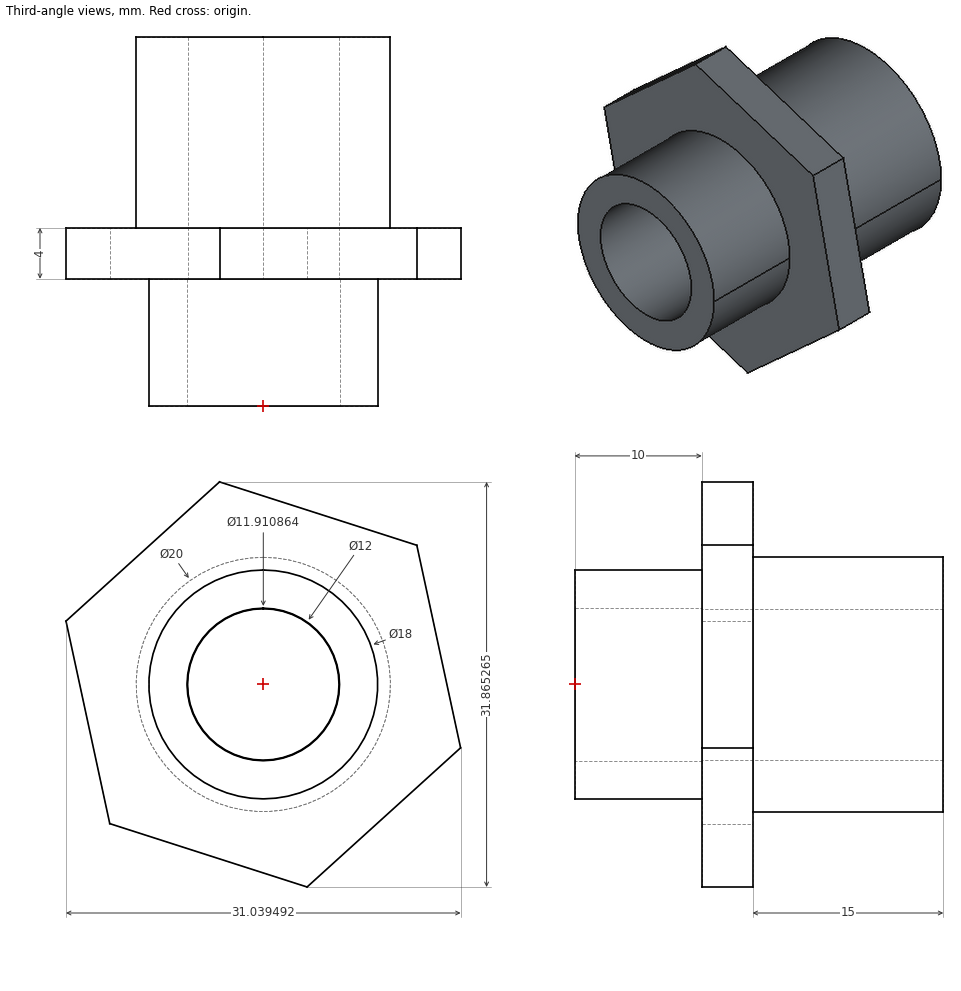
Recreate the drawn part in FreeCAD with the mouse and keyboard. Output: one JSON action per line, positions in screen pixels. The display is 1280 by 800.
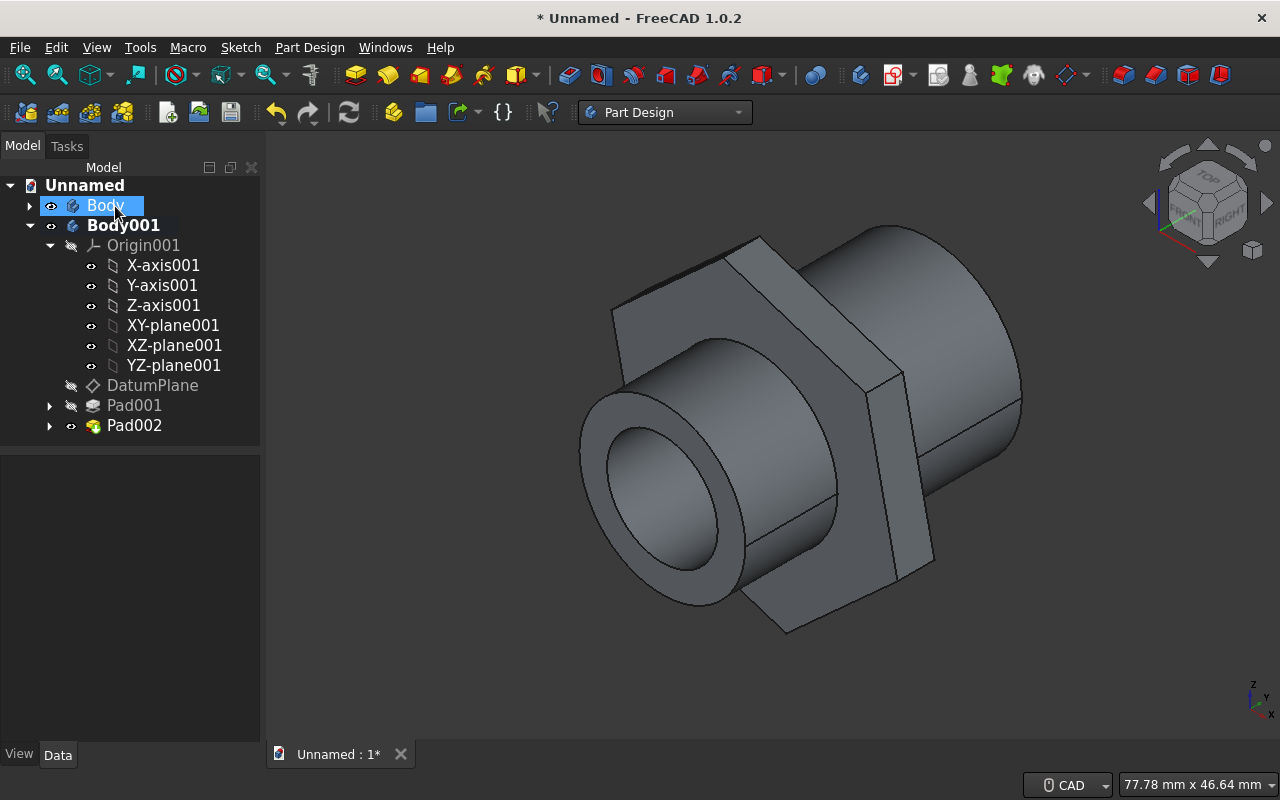
{"action": "left_click", "coordinate": [26, 76]}